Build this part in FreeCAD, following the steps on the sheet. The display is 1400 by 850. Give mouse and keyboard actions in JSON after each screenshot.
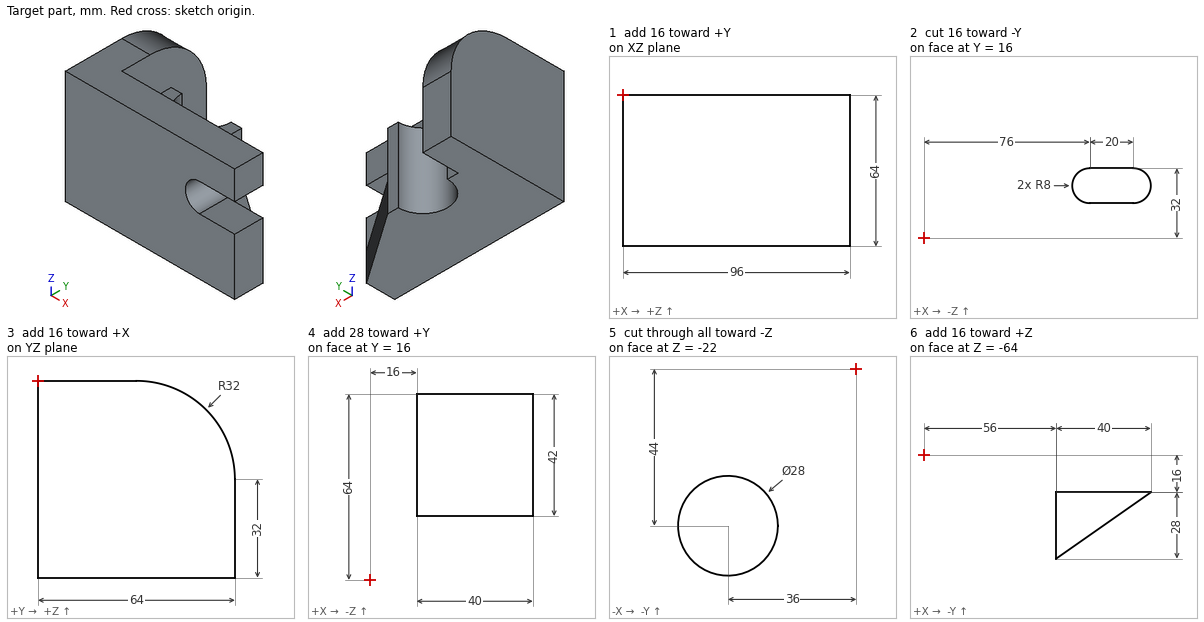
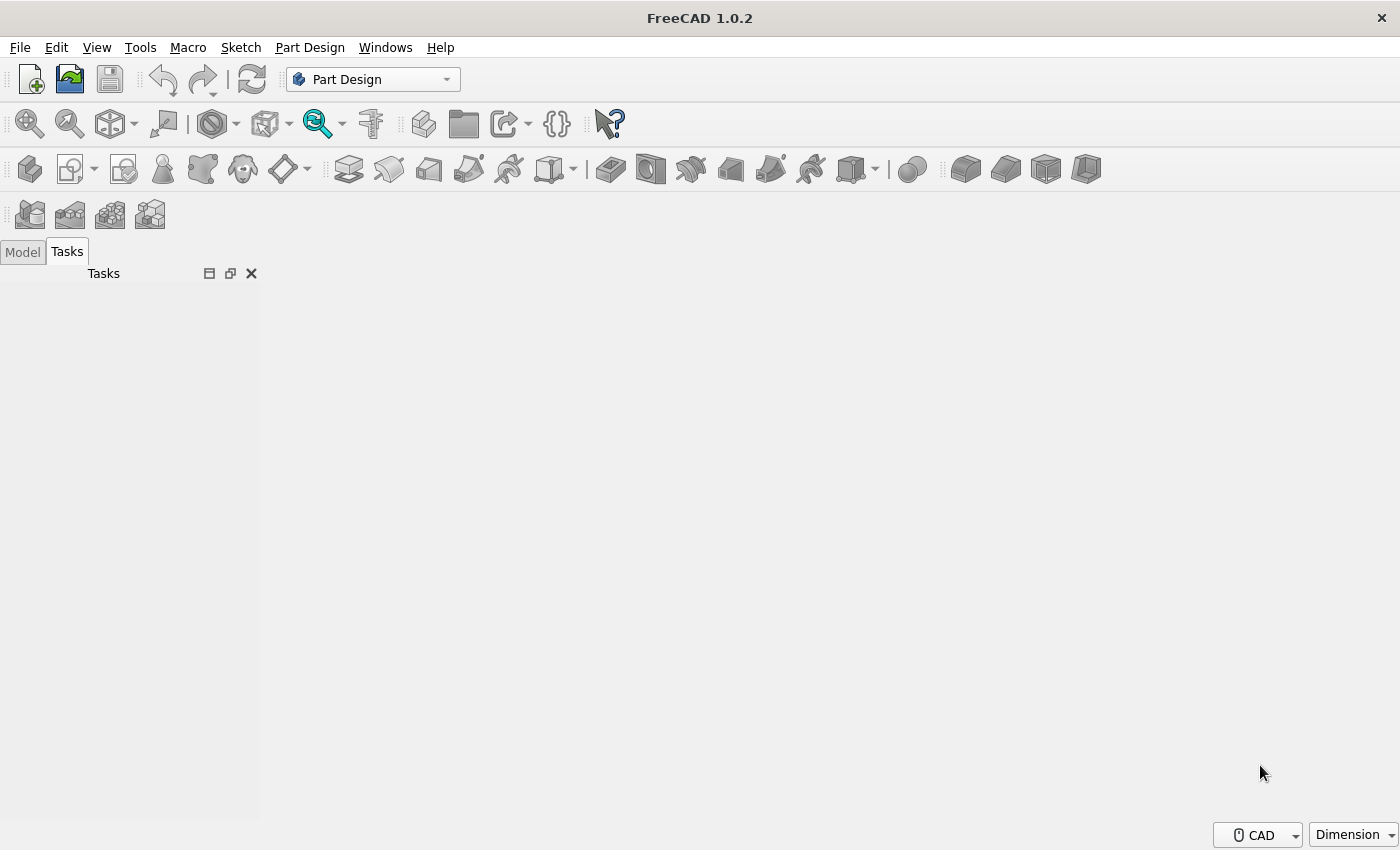
{"action": "left_click", "coordinate": [30, 80]}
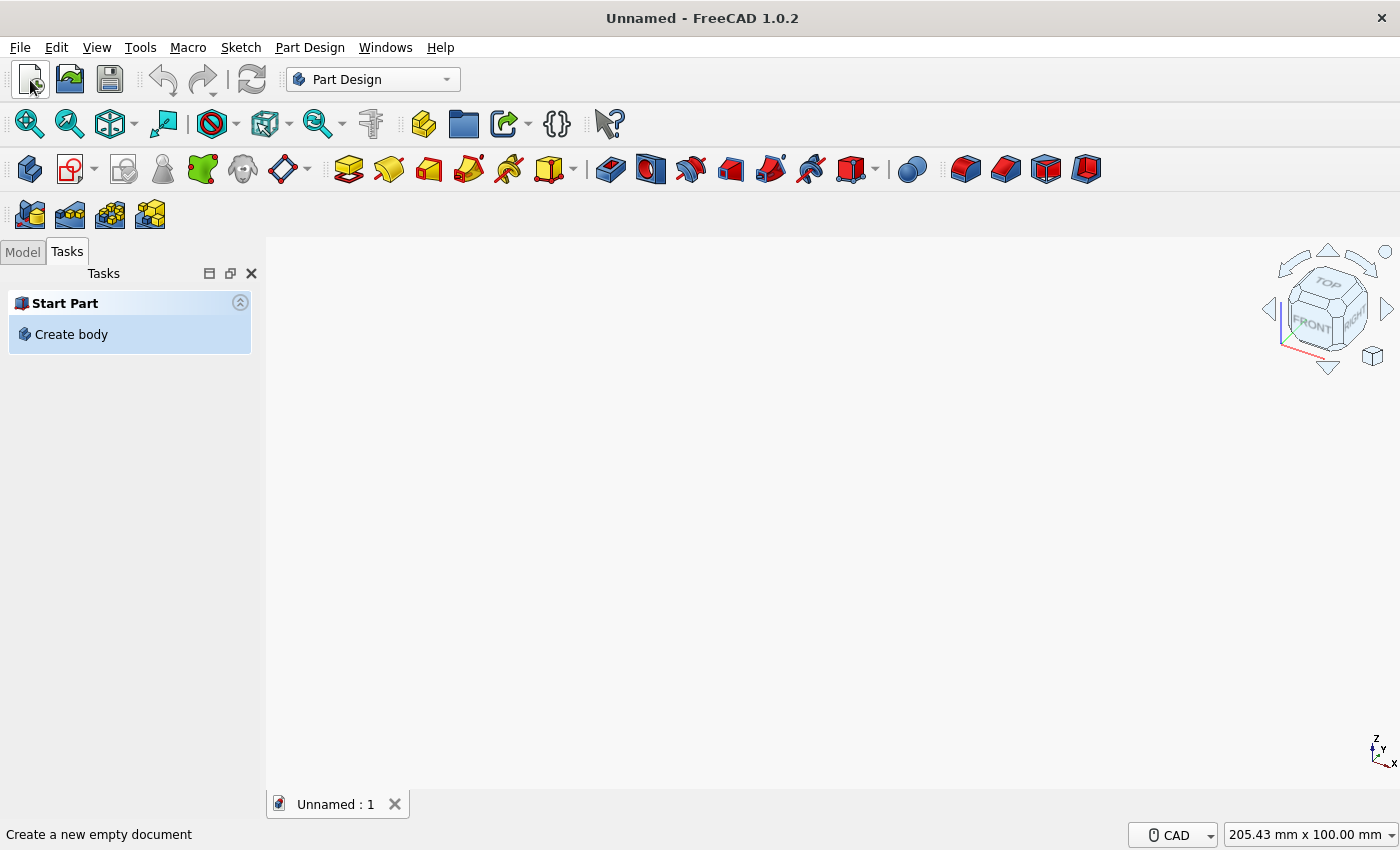
{"action": "left_click", "coordinate": [70, 170]}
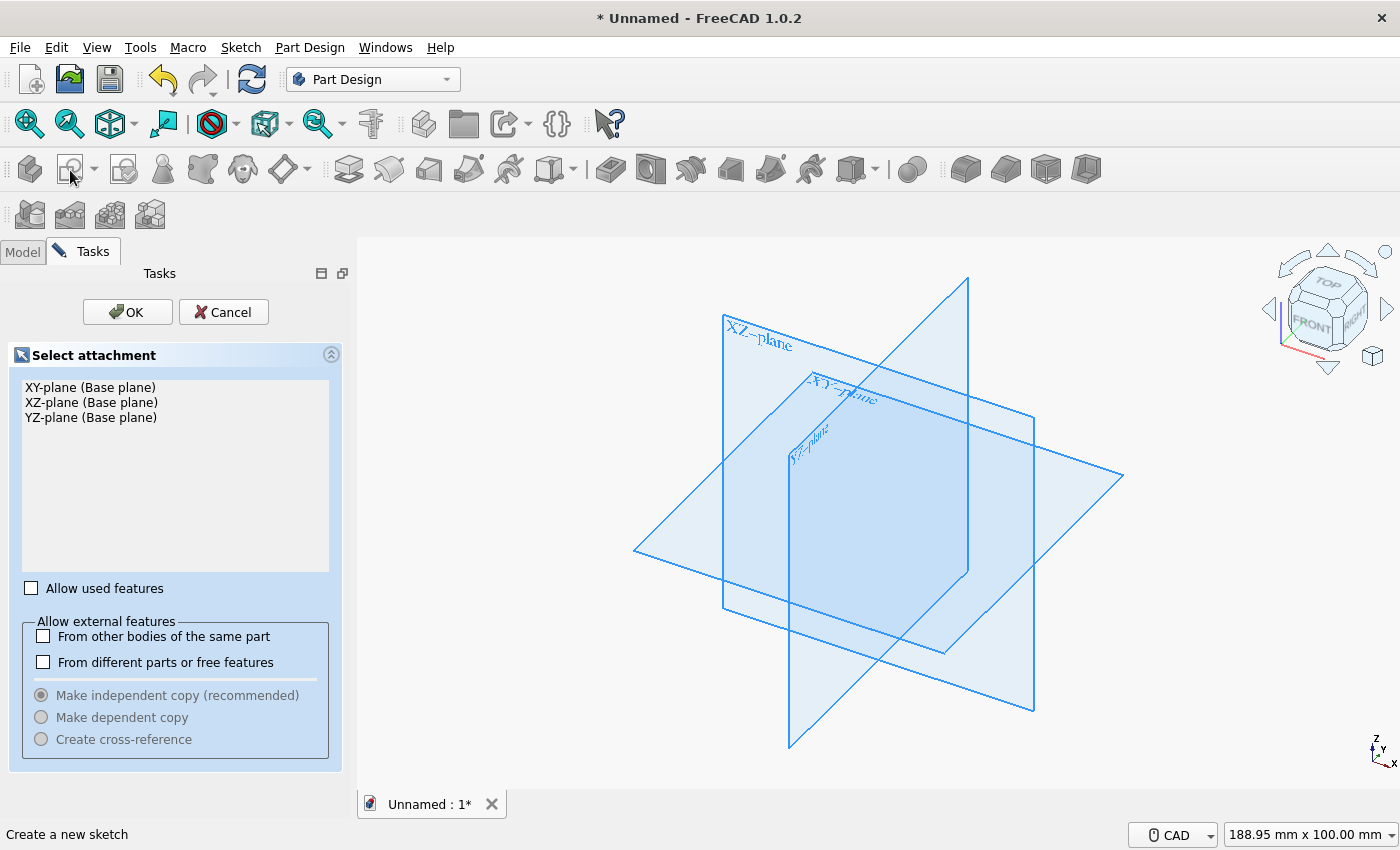
{"action": "left_click", "coordinate": [82, 402]}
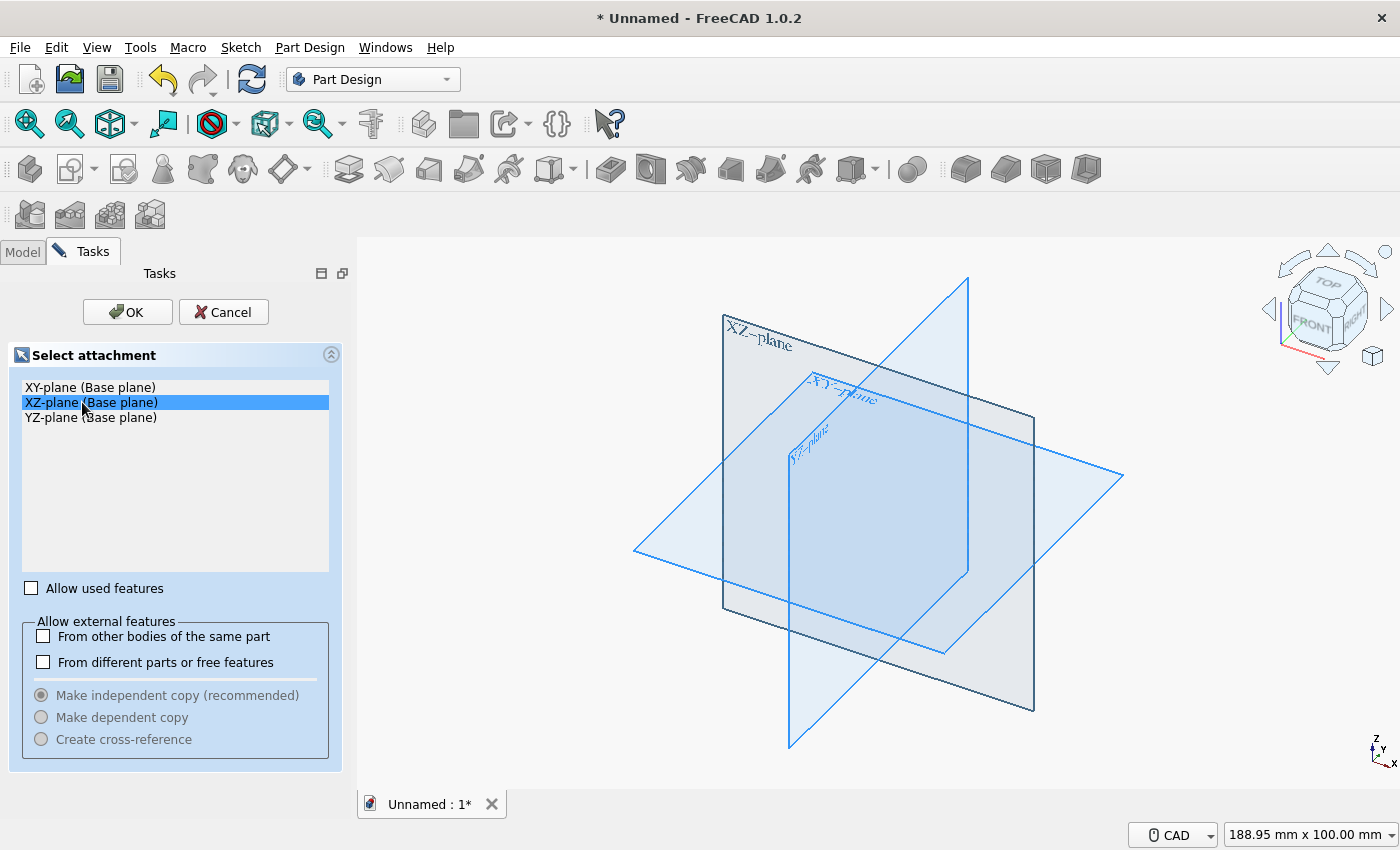
{"action": "left_click", "coordinate": [128, 312]}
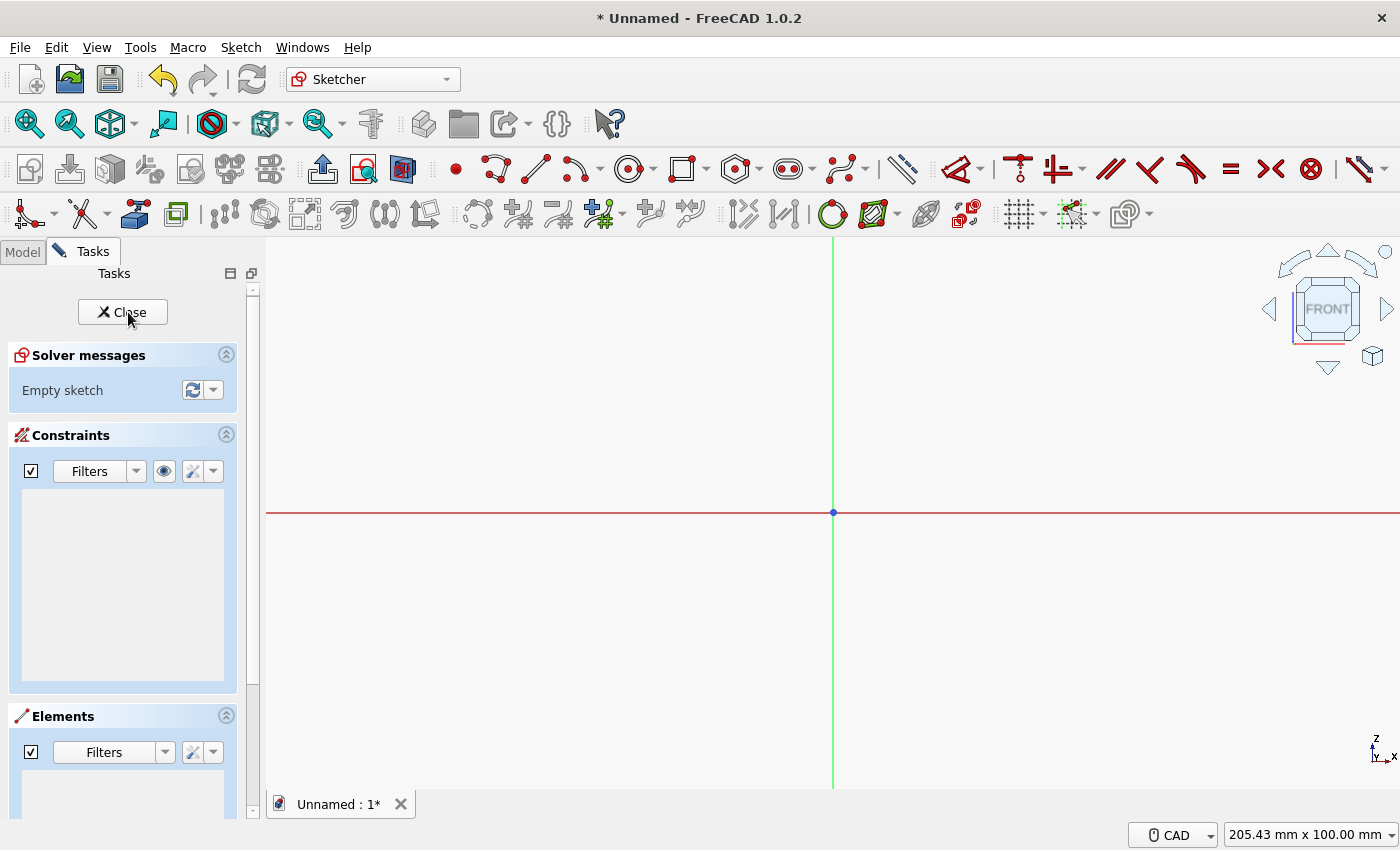
{"action": "scroll", "coordinate": [294, 265], "scroll_direction": "down", "scroll_amount": 2}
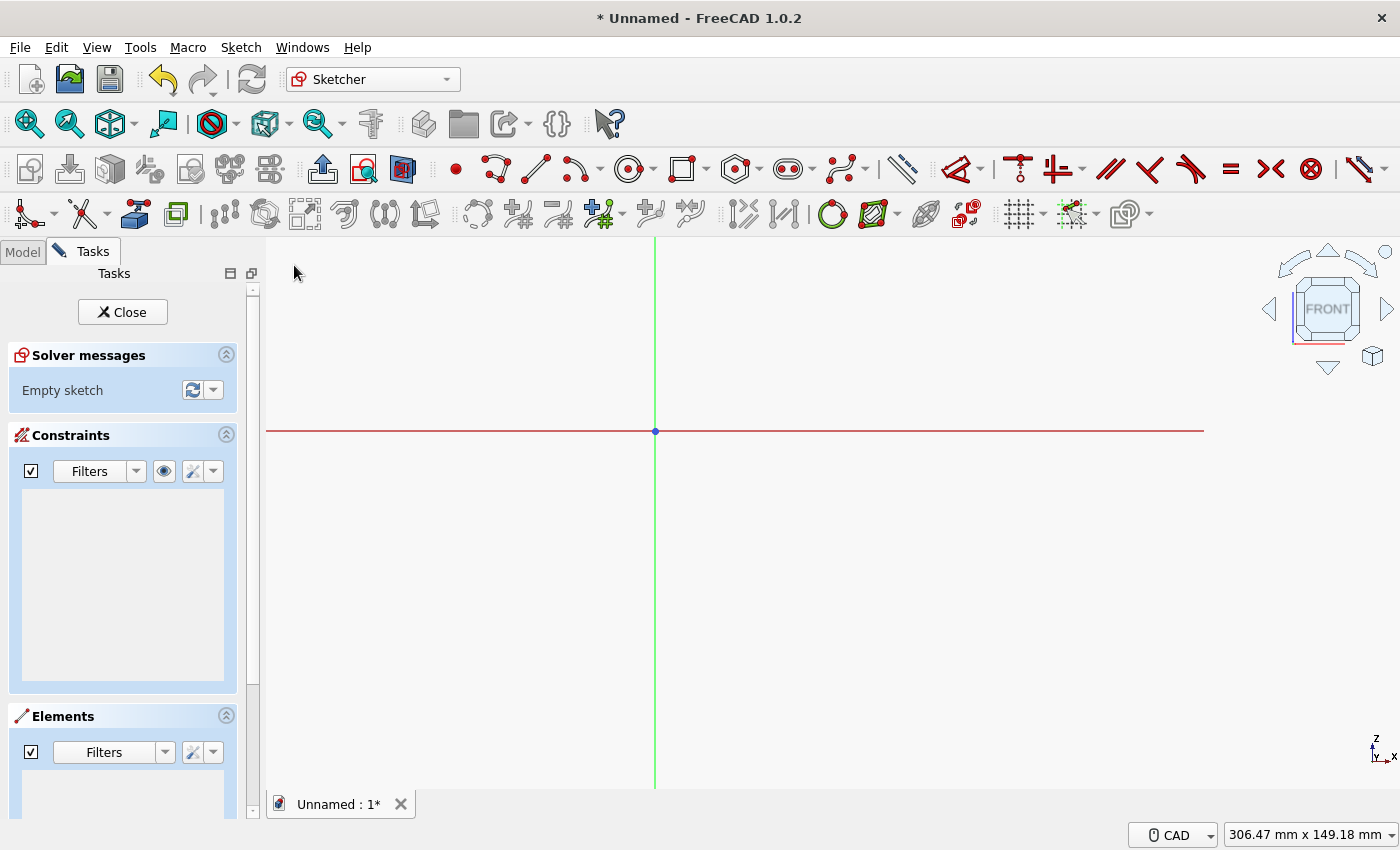
{"action": "scroll", "coordinate": [972, 624], "scroll_direction": "up", "scroll_amount": 2}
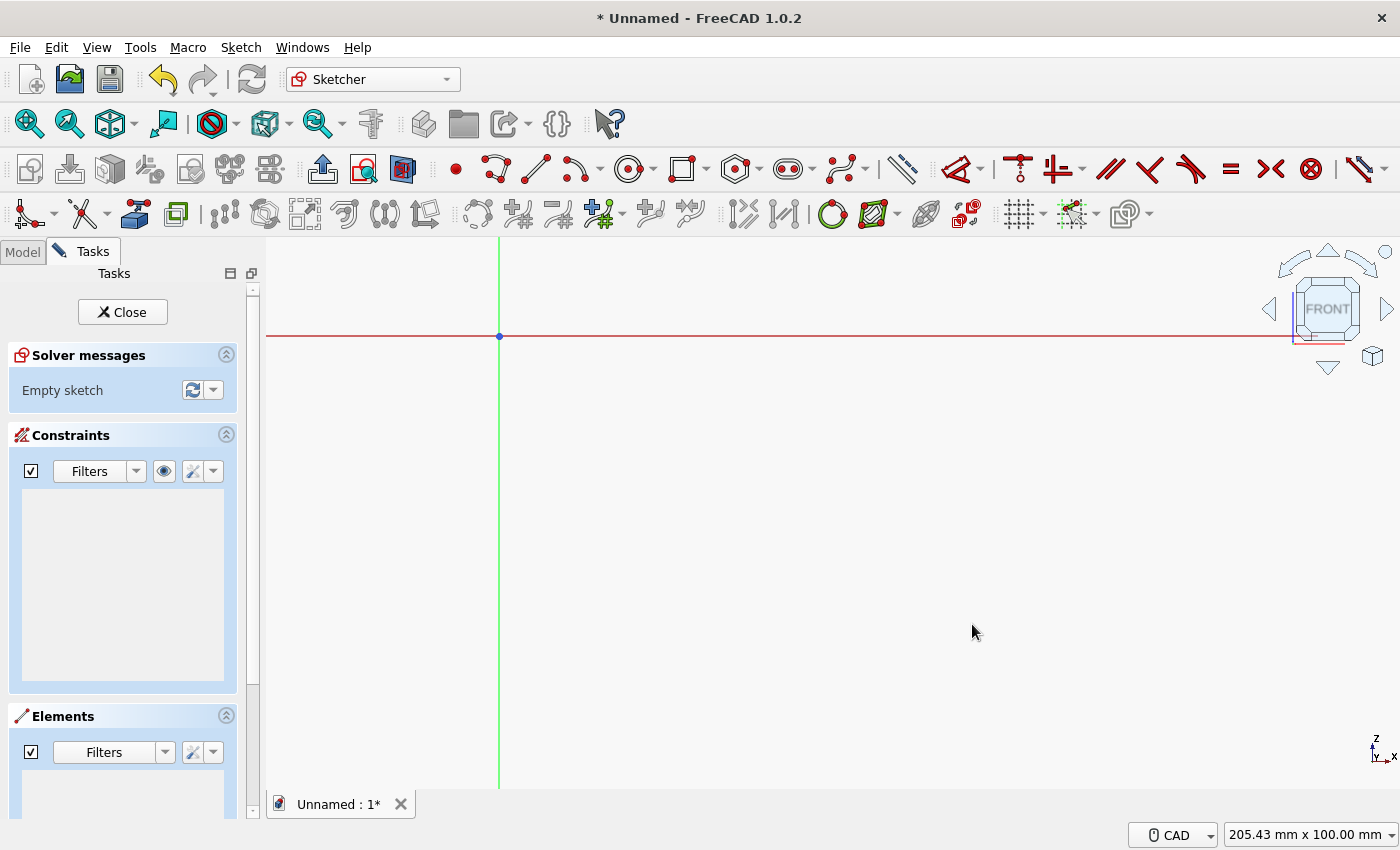
{"action": "left_click", "coordinate": [682, 170]}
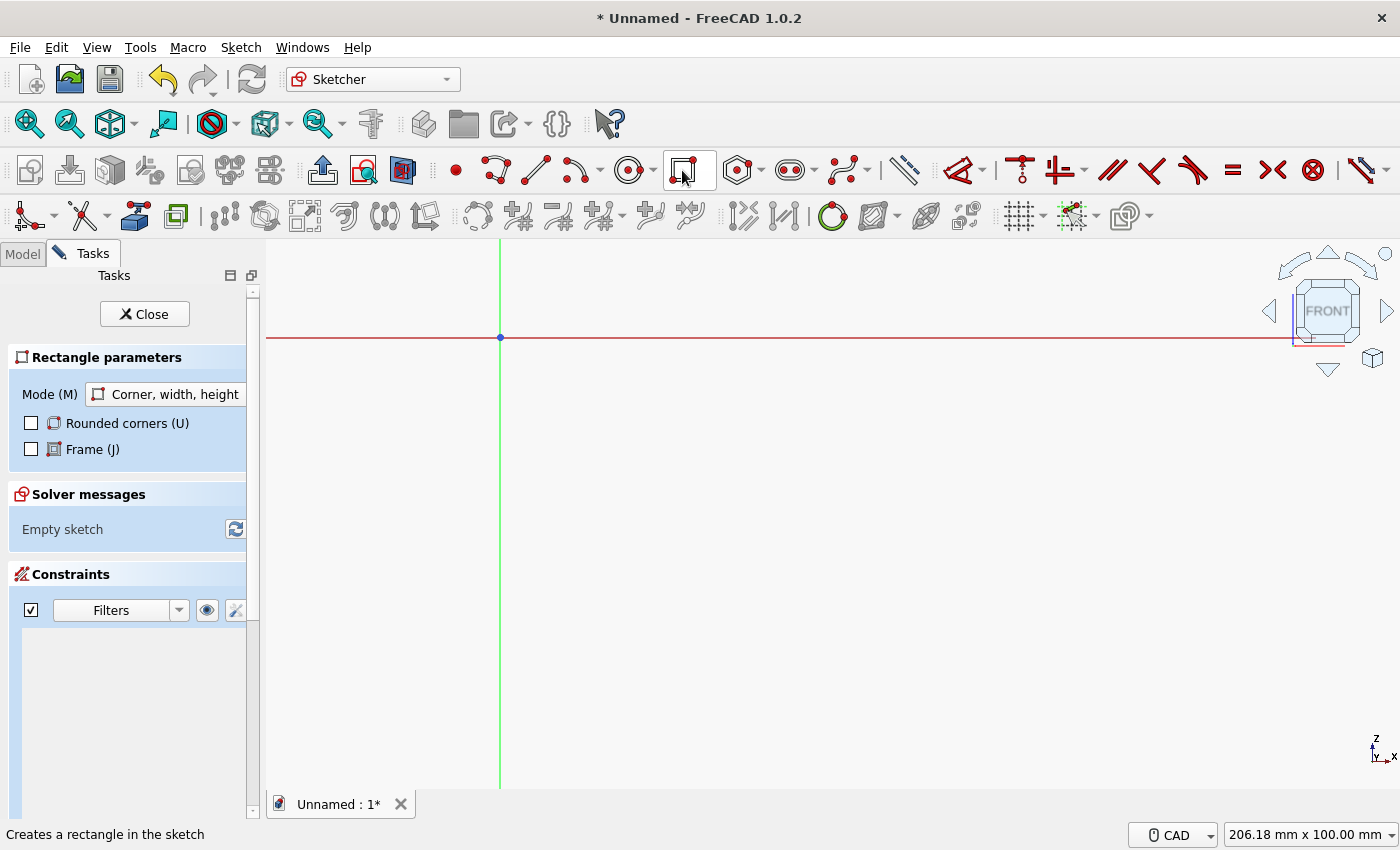
{"action": "left_click", "coordinate": [500, 338]}
{"action": "mouse_move", "coordinate": [1028, 690]}